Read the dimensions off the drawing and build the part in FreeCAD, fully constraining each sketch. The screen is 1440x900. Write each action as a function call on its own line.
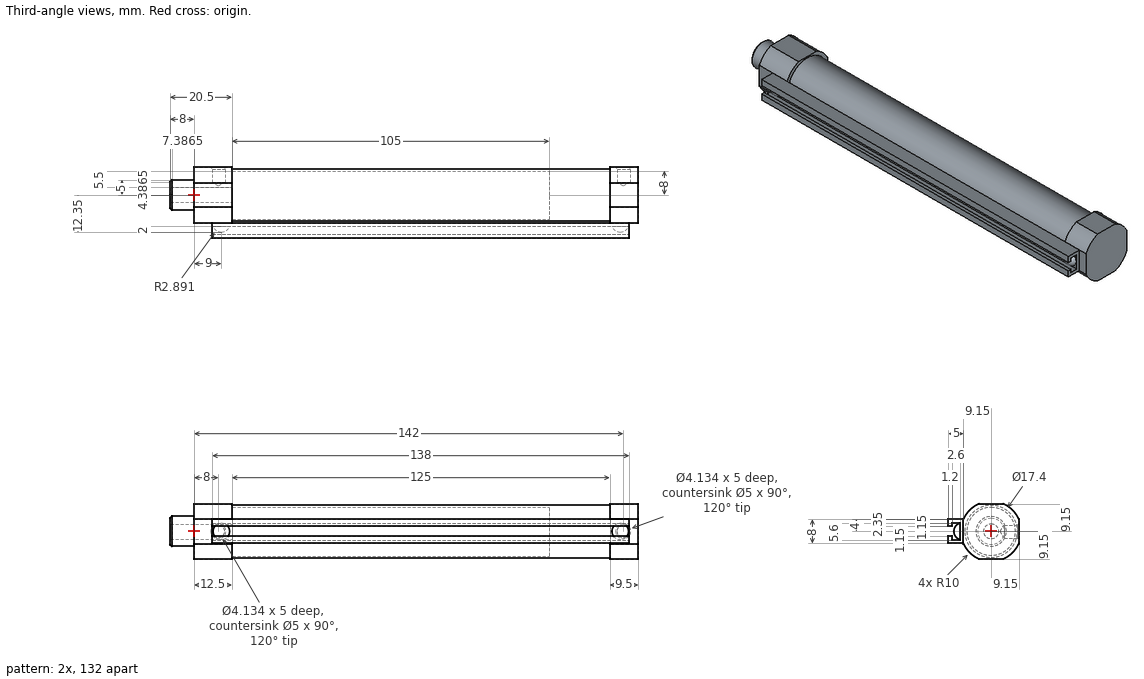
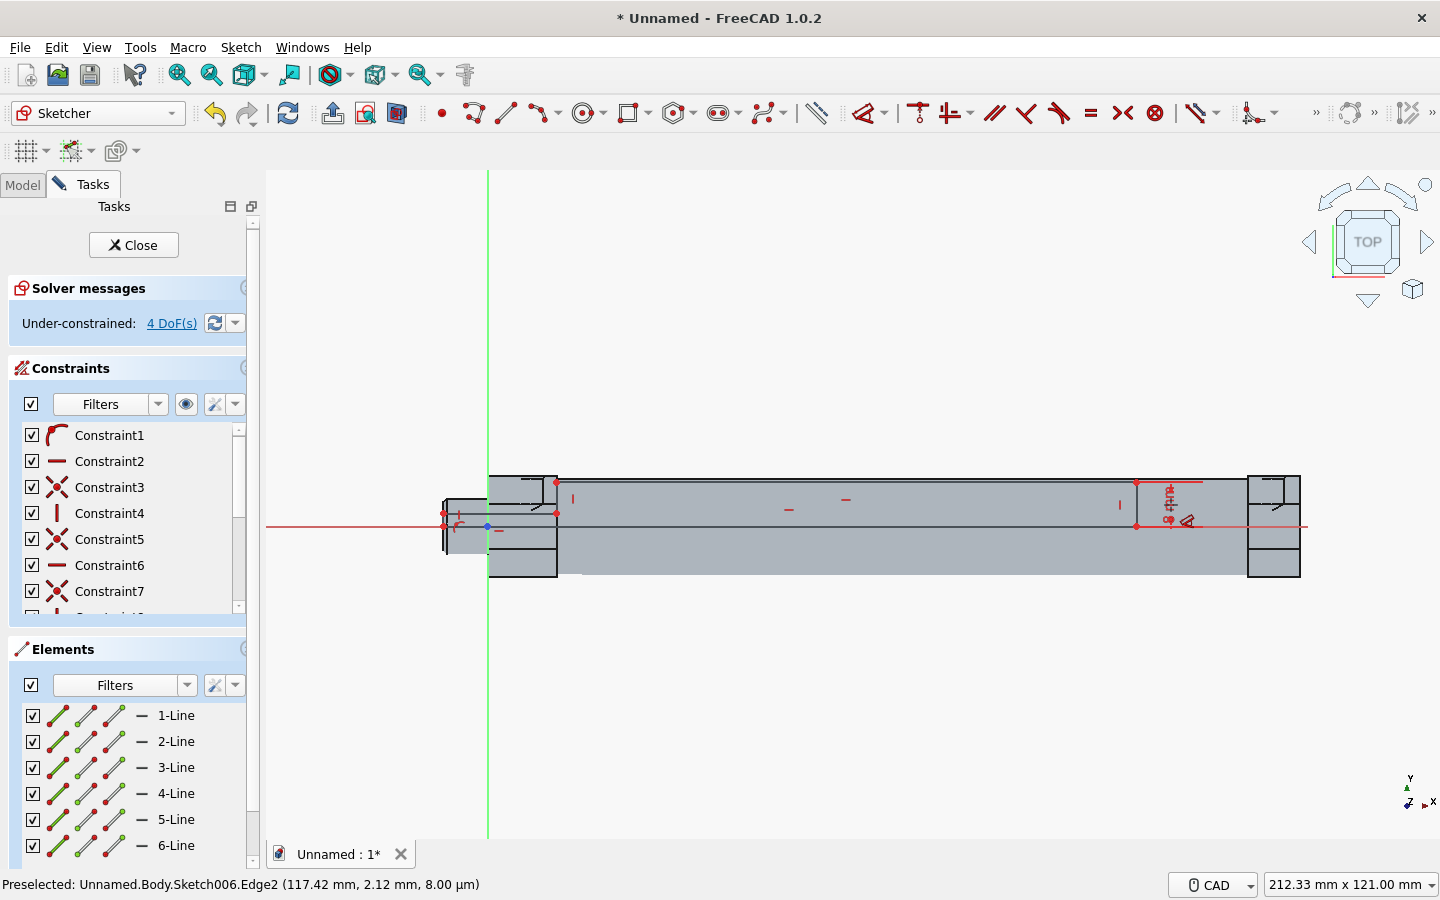
click(443, 527)
click(465, 561)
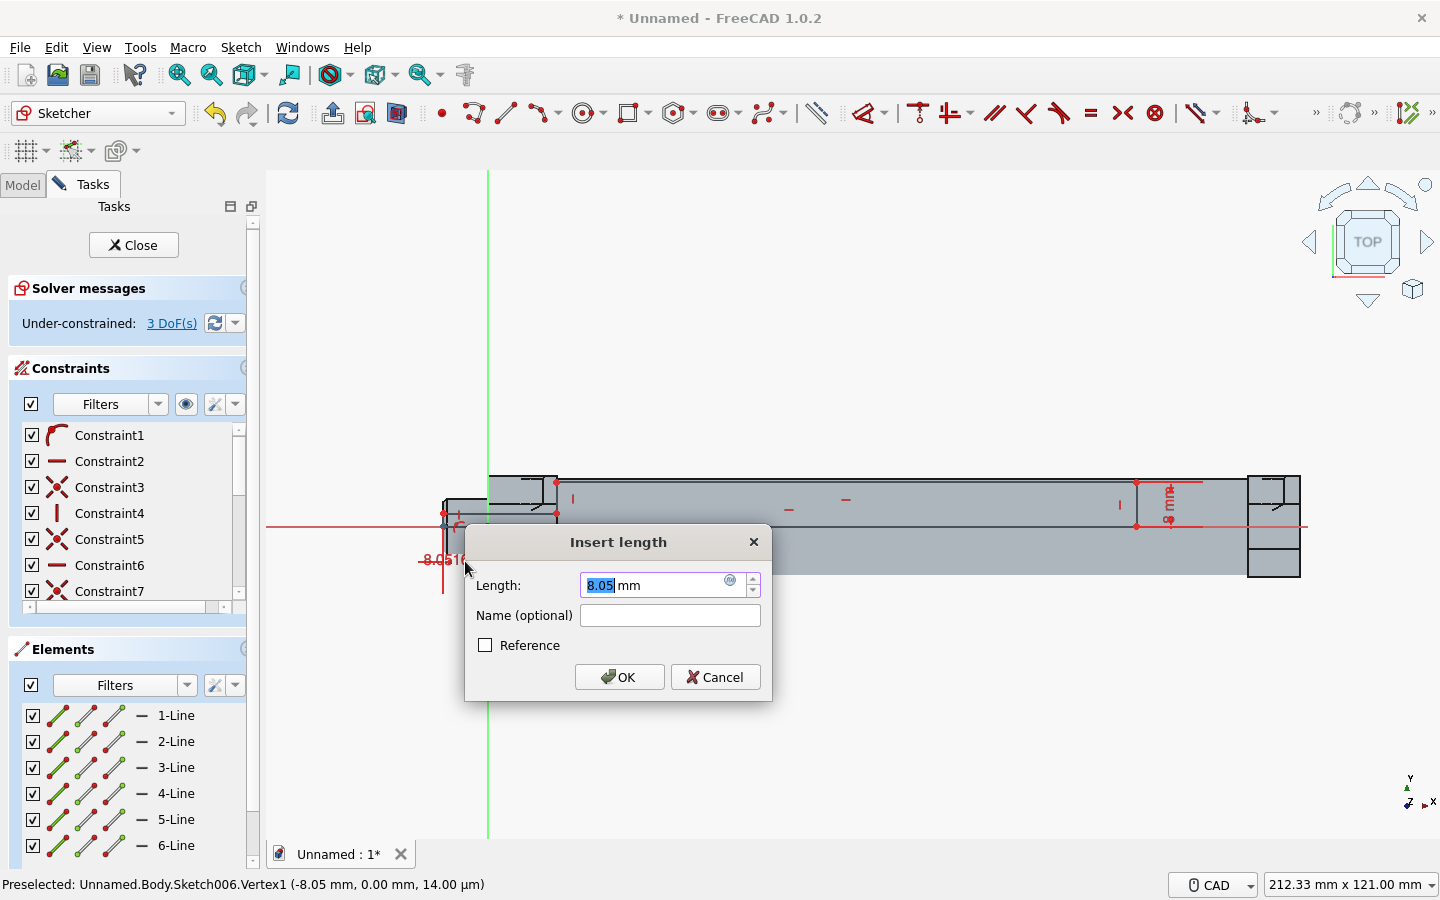
text(8)
key(Return)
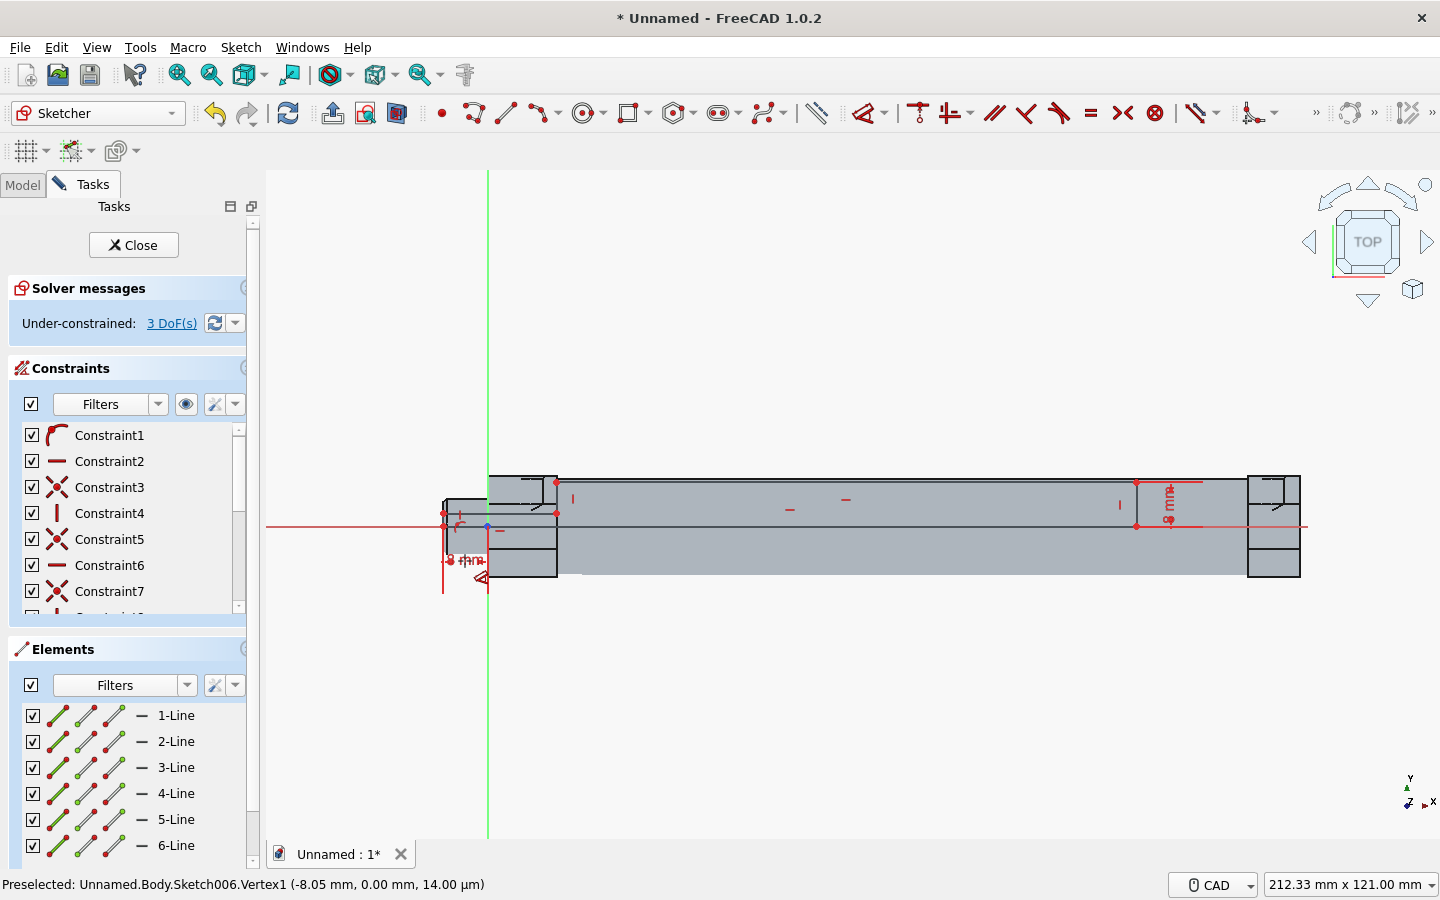
click(963, 482)
click(847, 448)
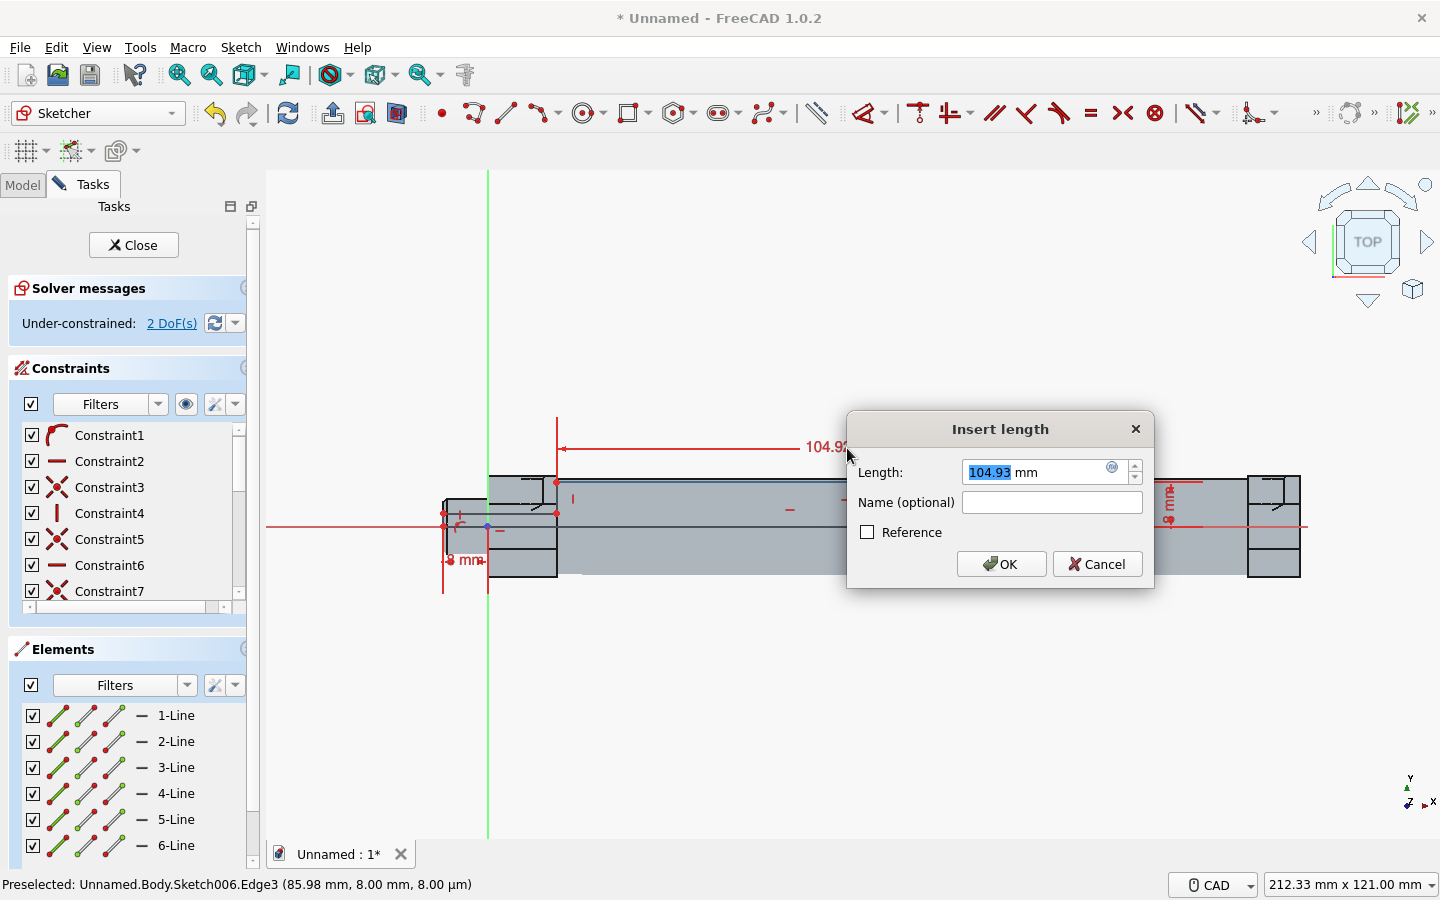
text(105)
key(Return)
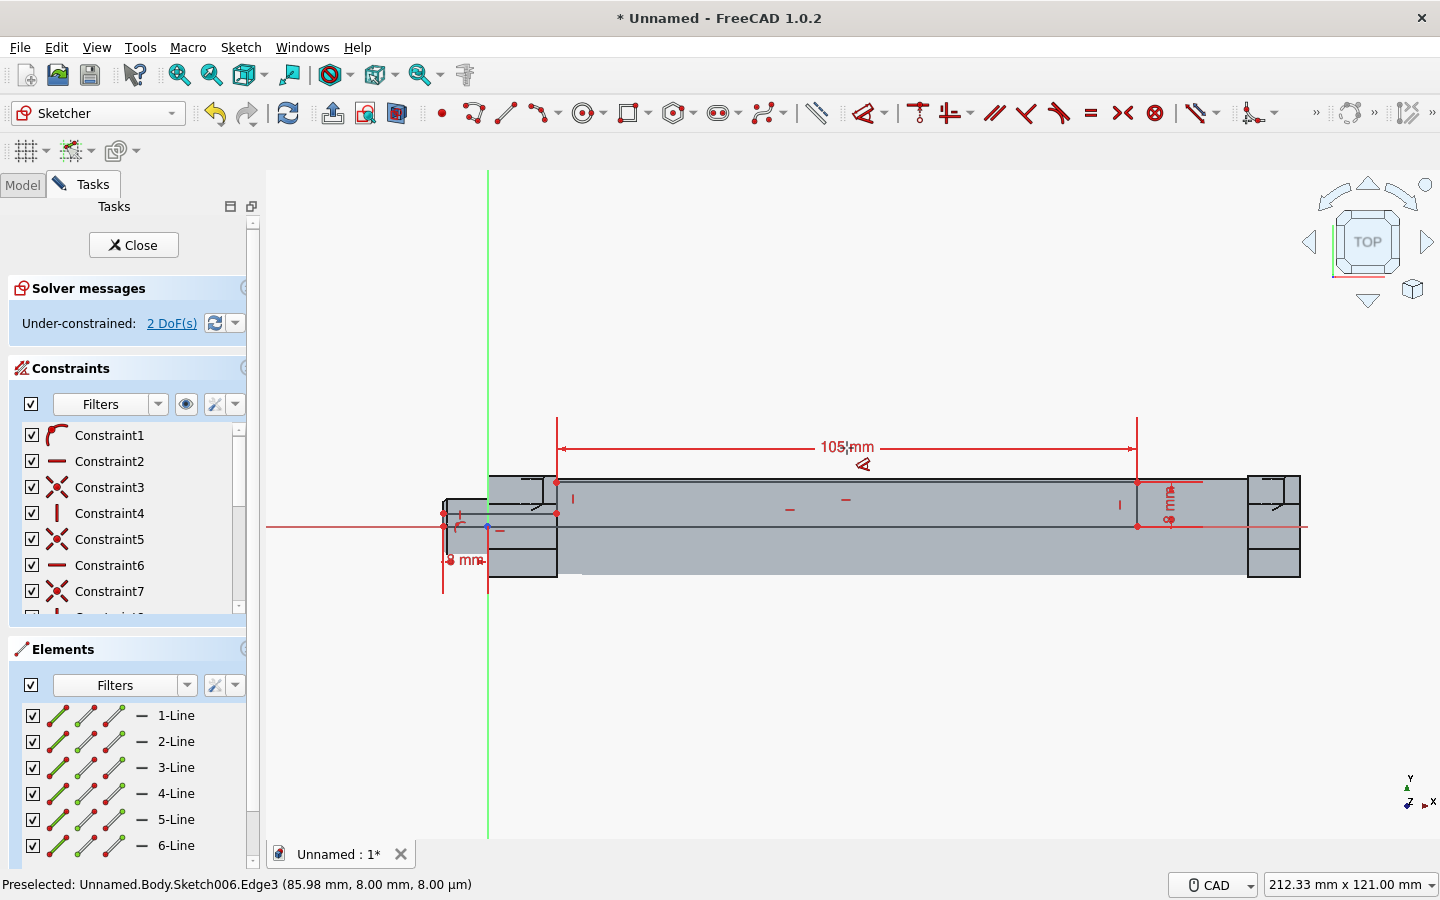
scroll(557, 492, up, 2)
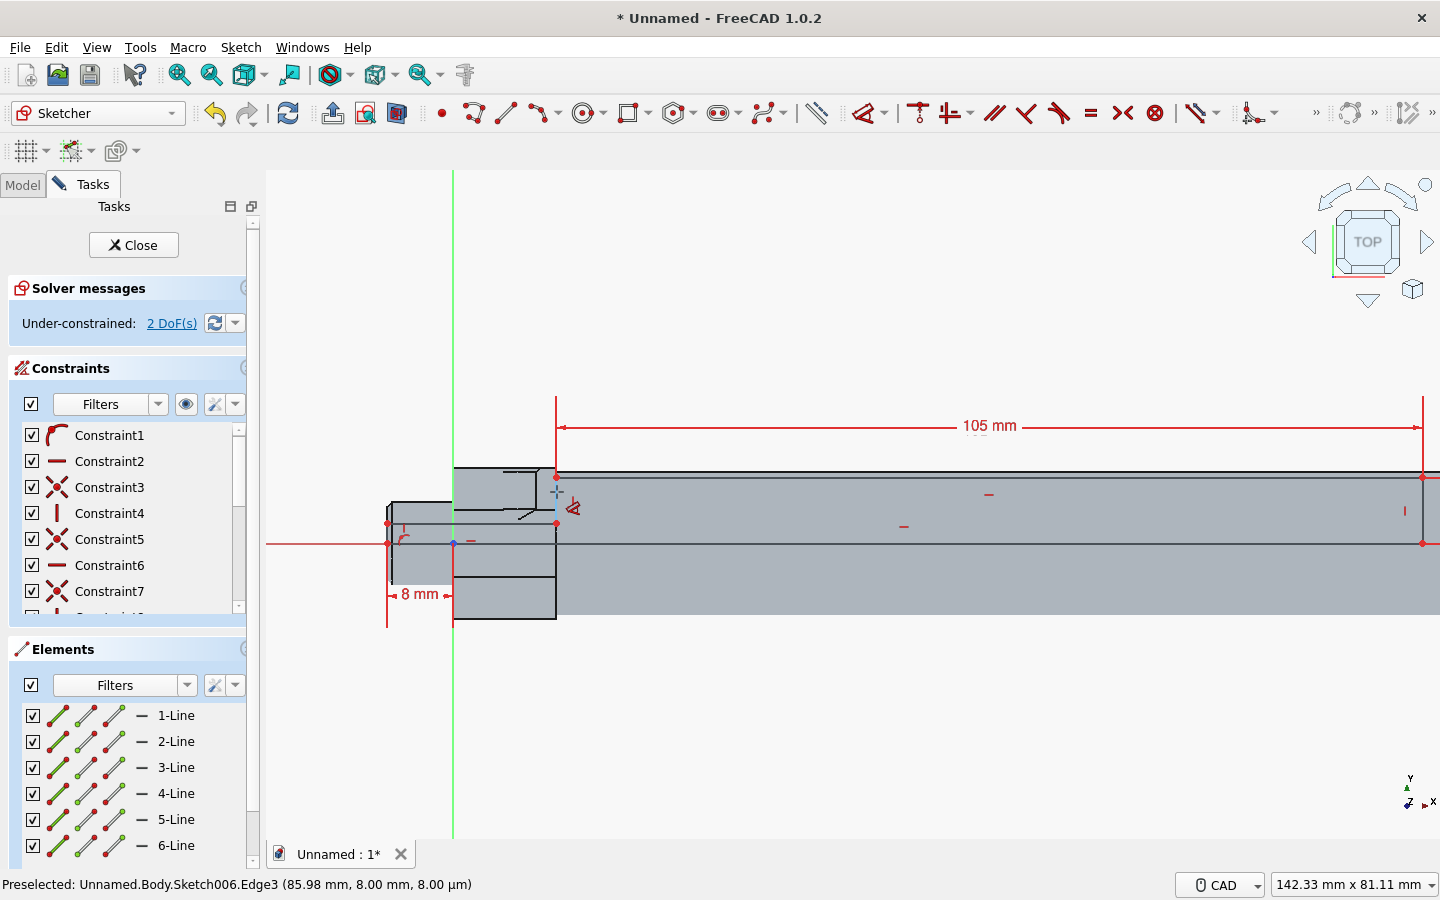
click(556, 491)
click(522, 501)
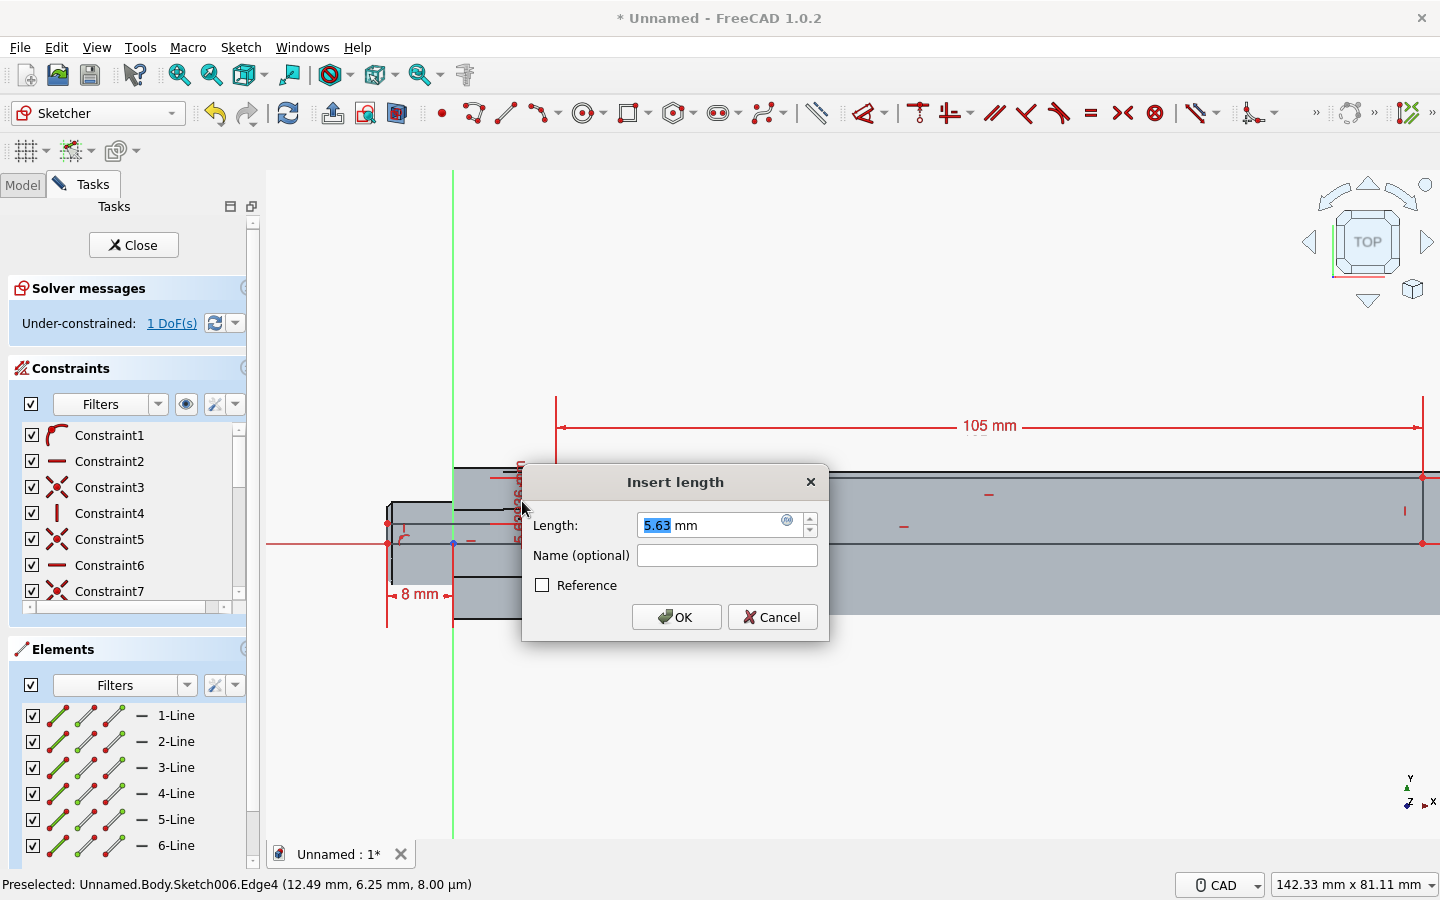
text(5.5)
key(Return)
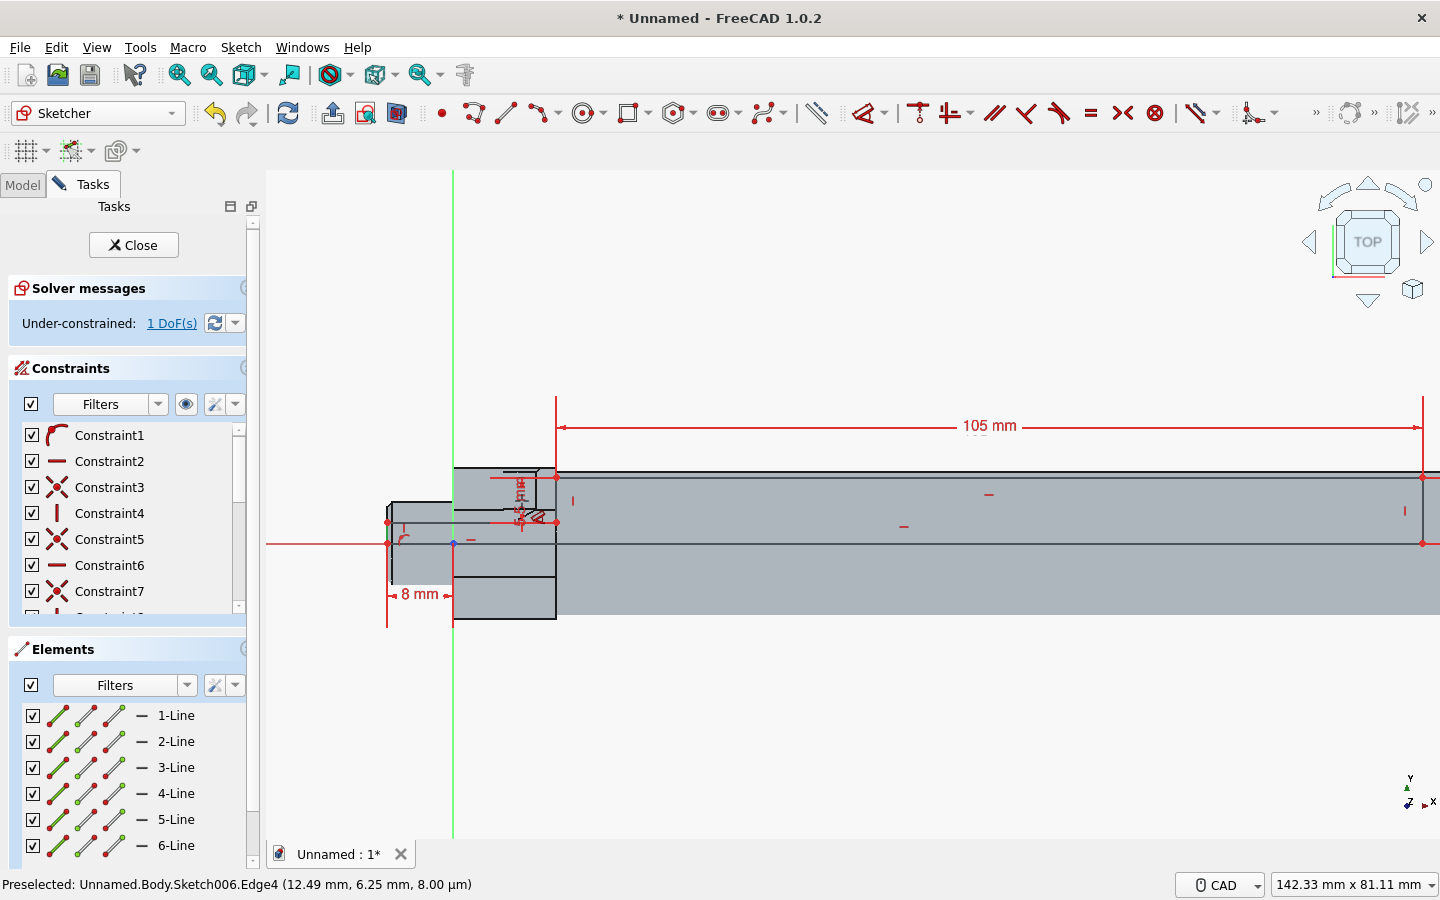
click(506, 523)
click(472, 557)